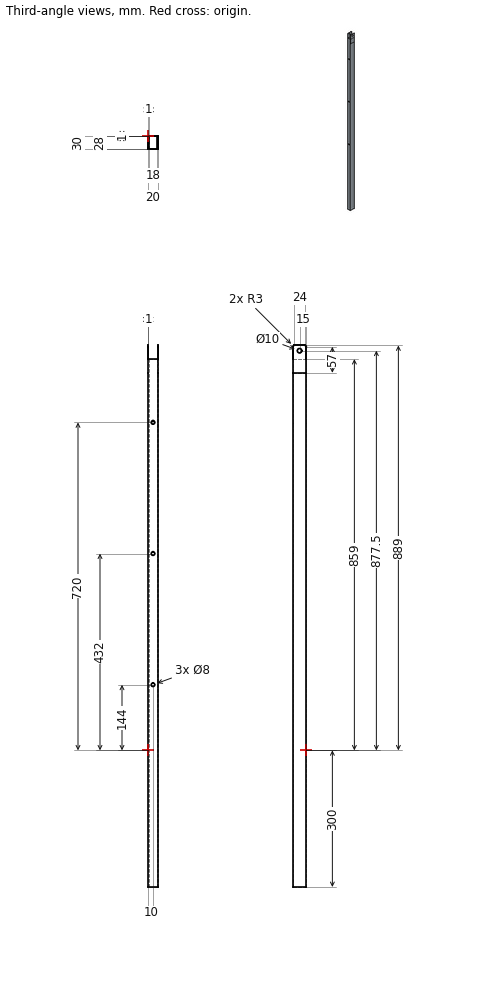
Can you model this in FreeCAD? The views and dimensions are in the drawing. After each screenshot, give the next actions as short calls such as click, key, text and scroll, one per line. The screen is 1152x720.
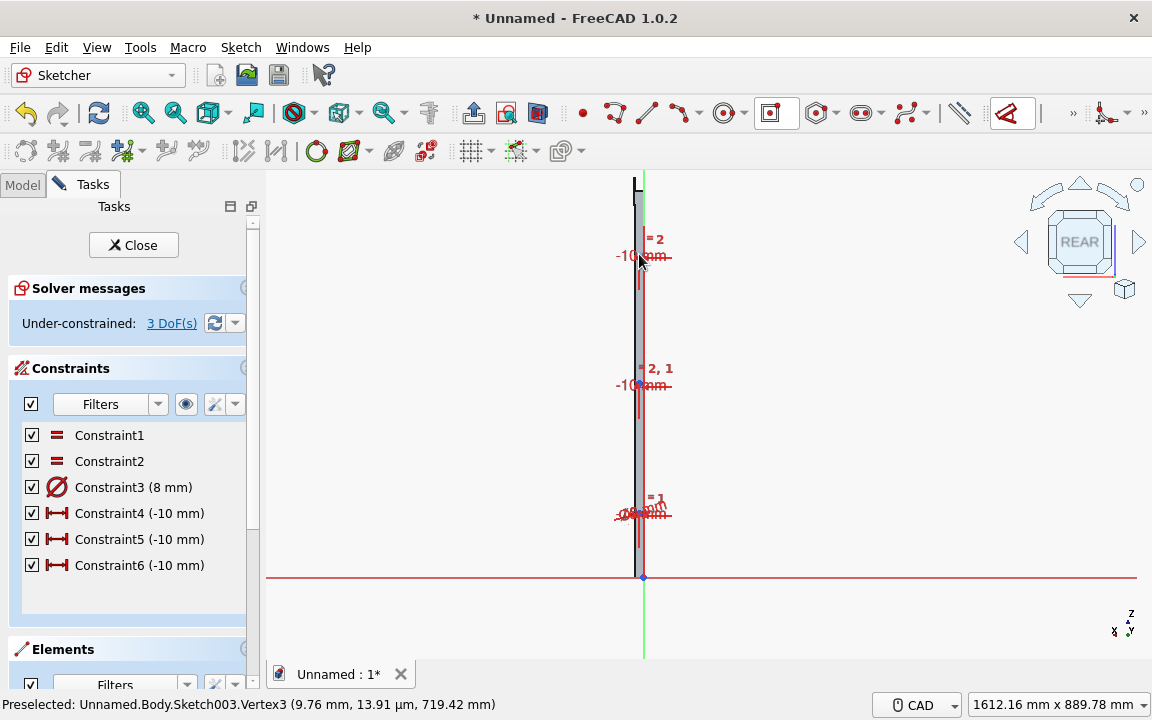
click(639, 513)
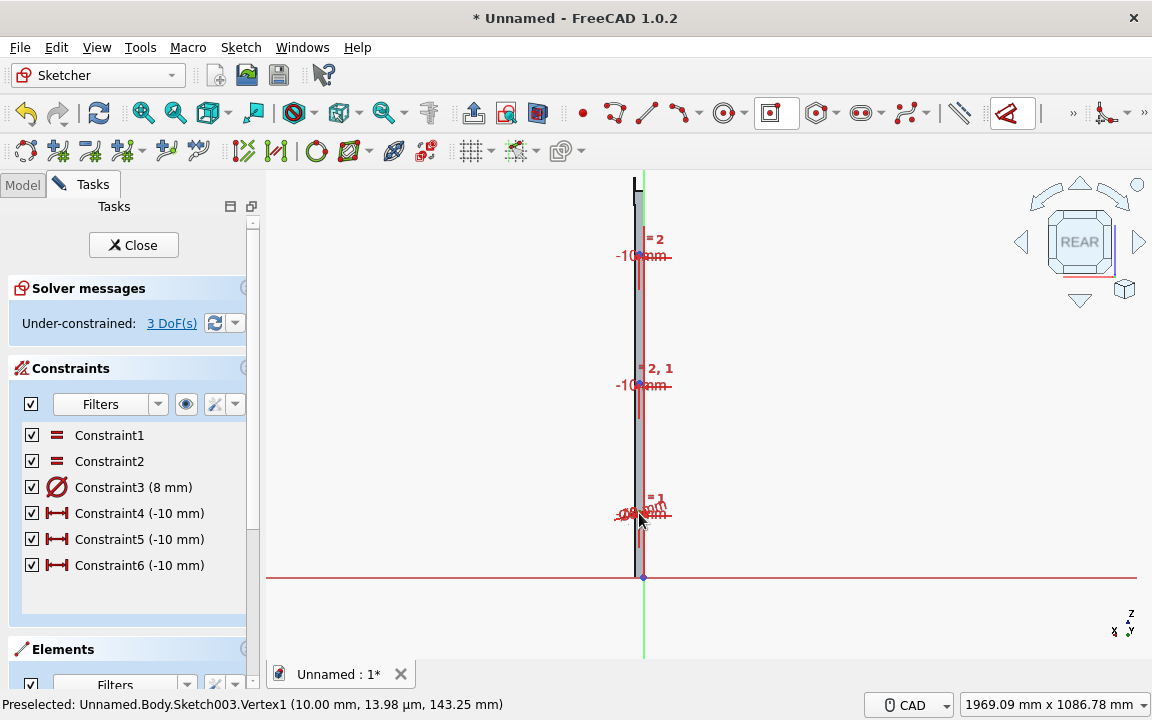
key(i)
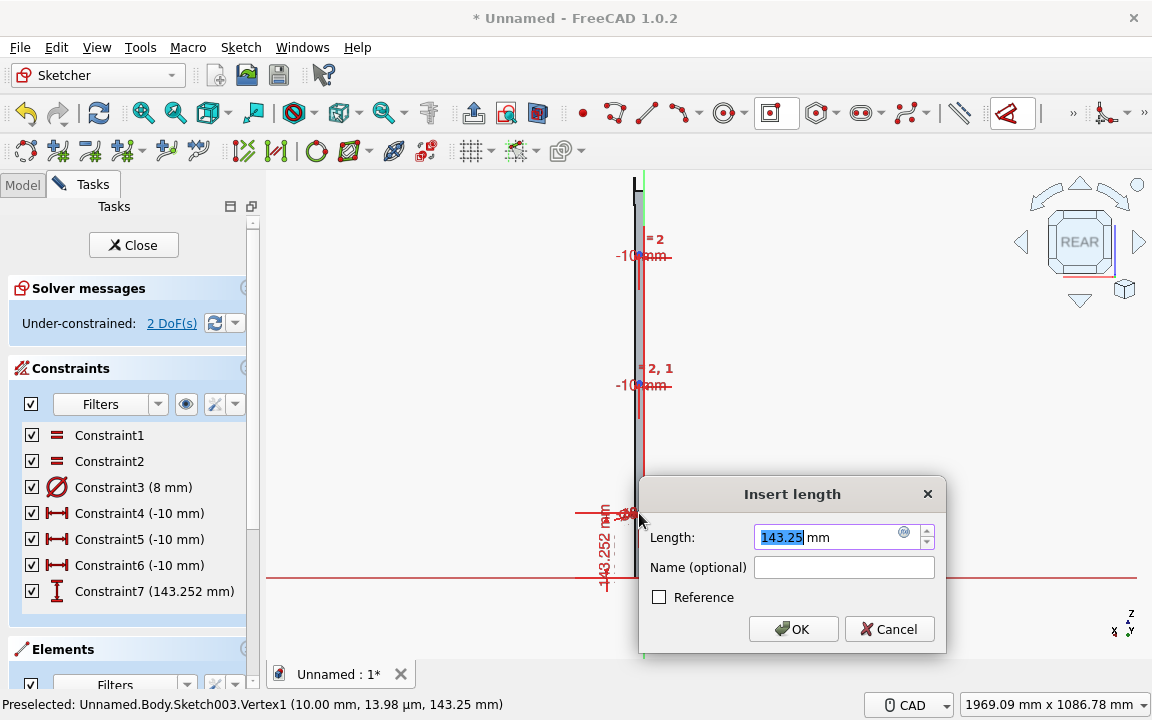
text(144)
key(Return)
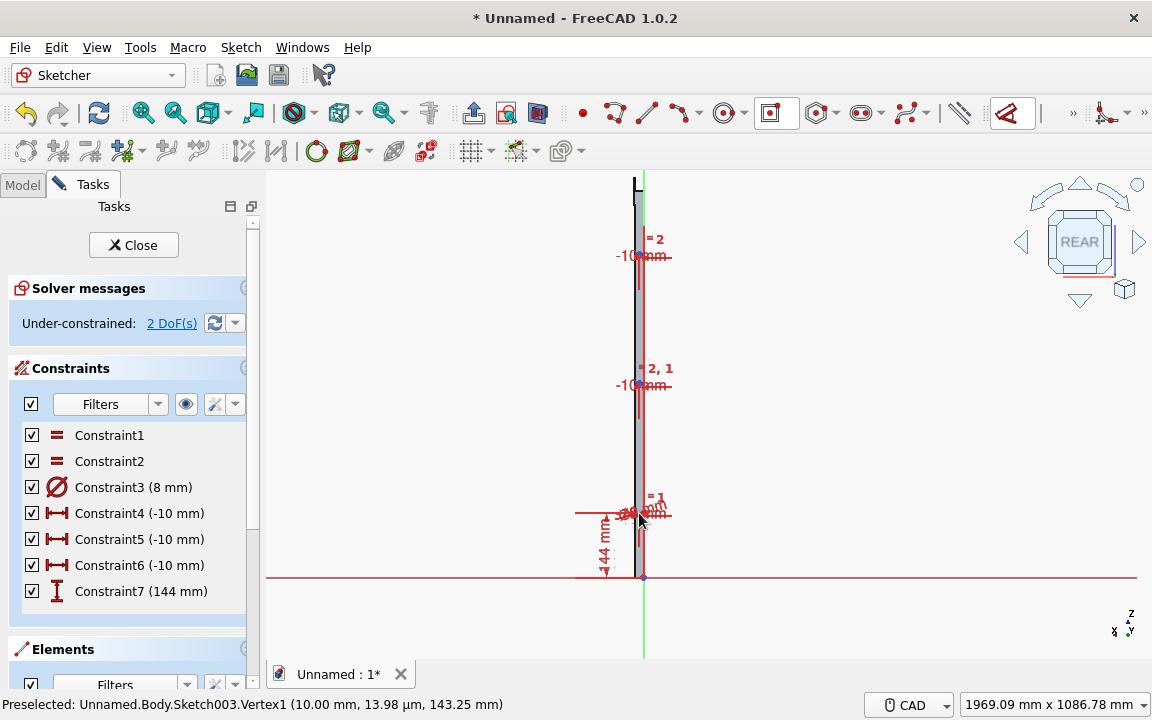
click(639, 384)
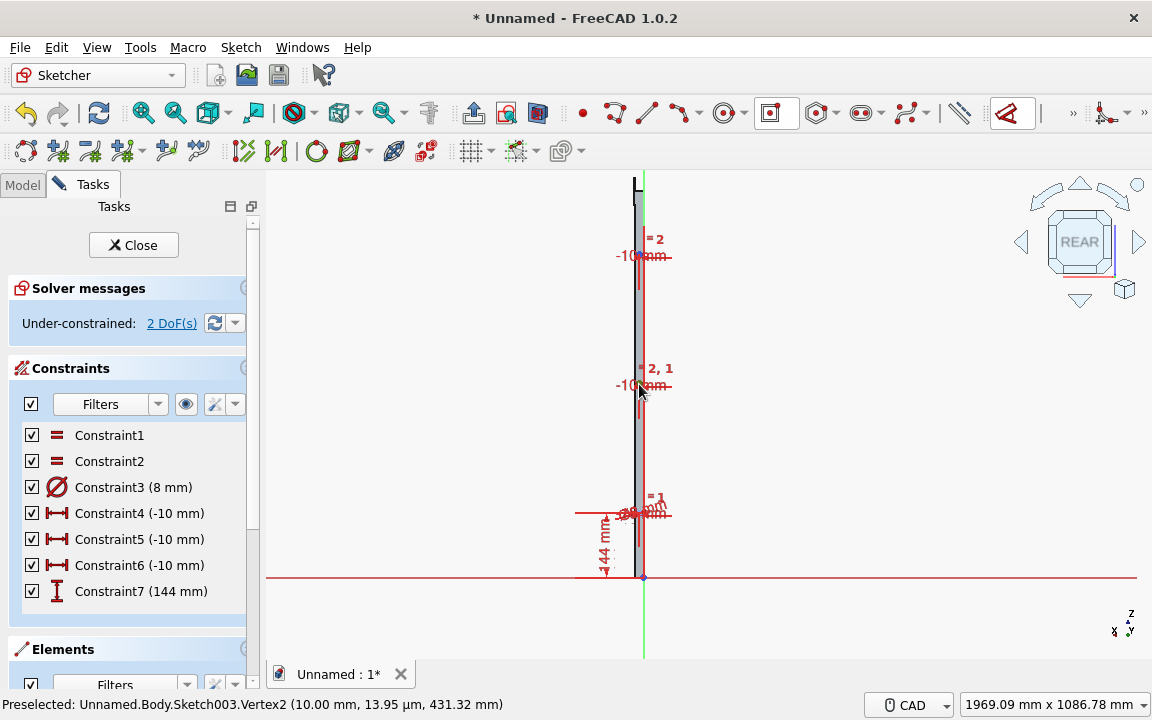
key(i)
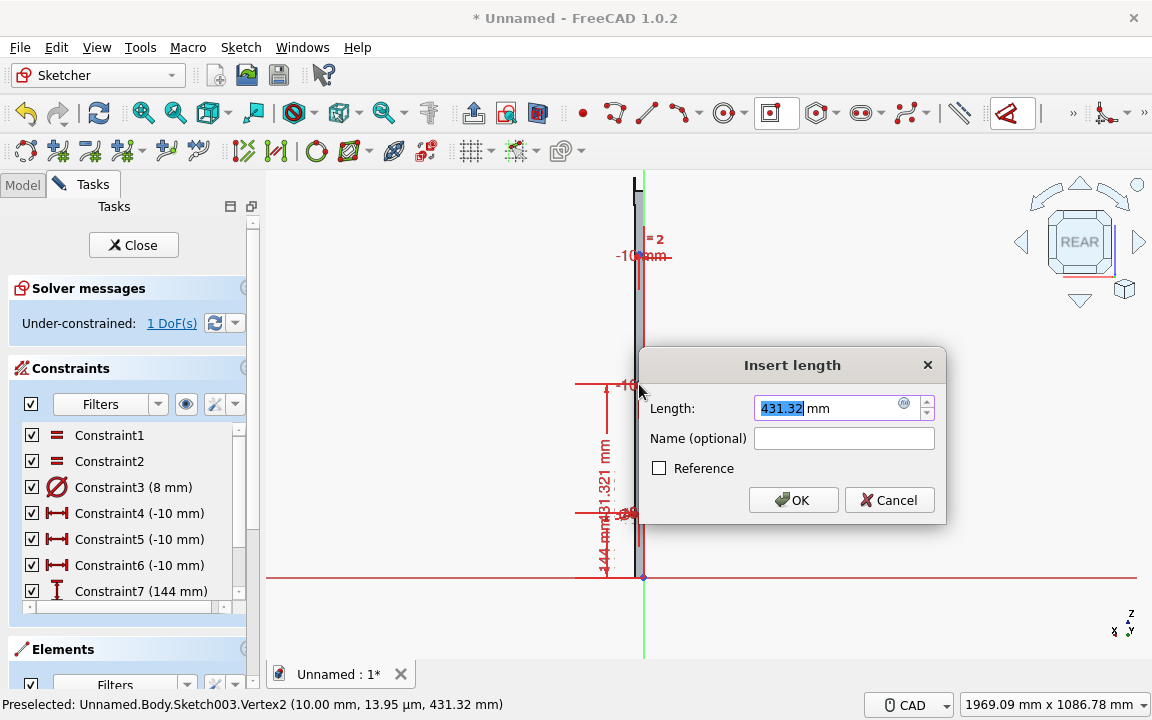
text(432)
key(Return)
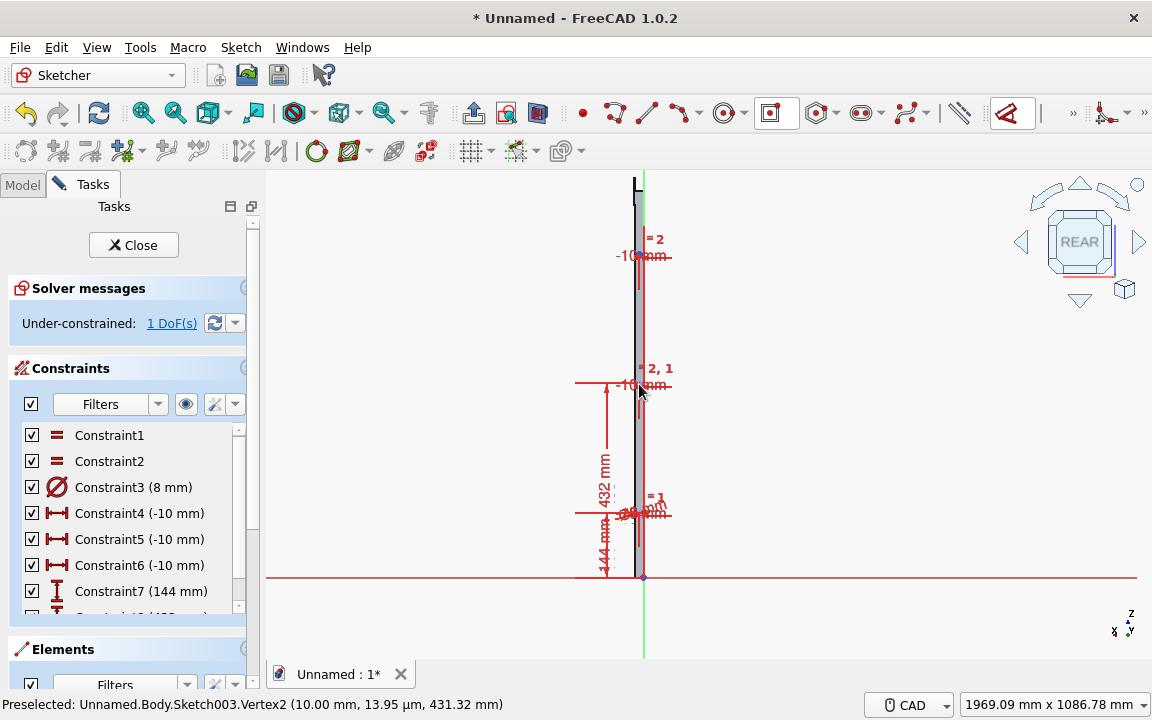
click(639, 254)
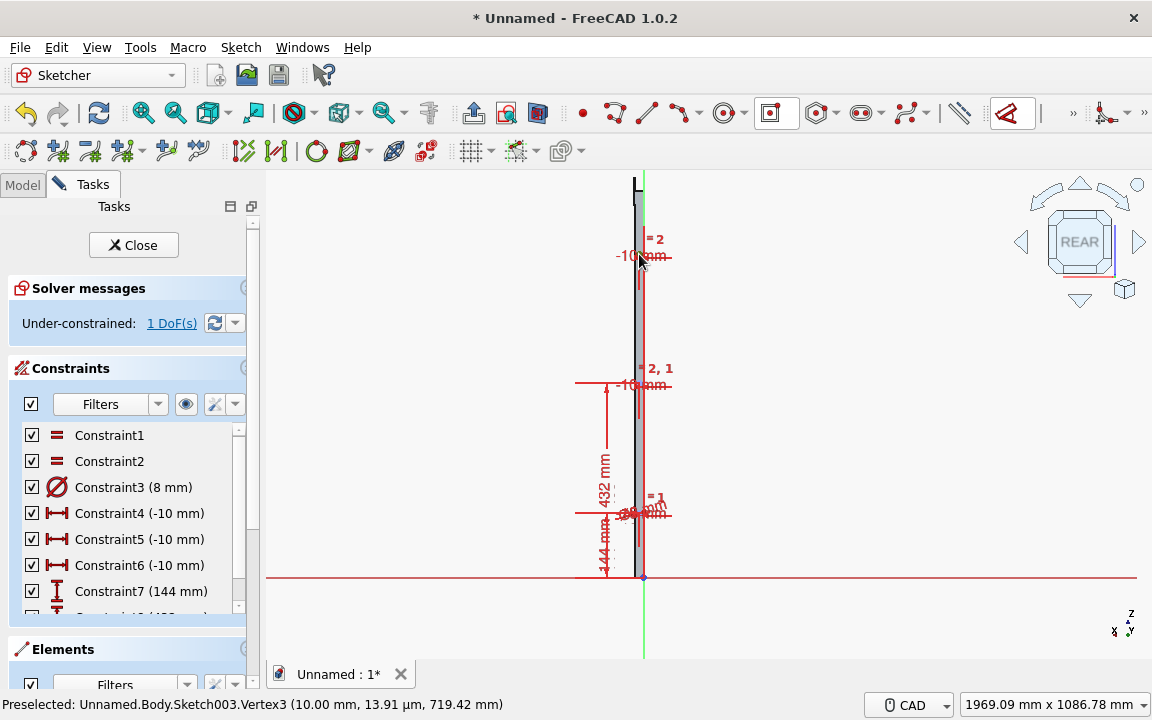
key(i)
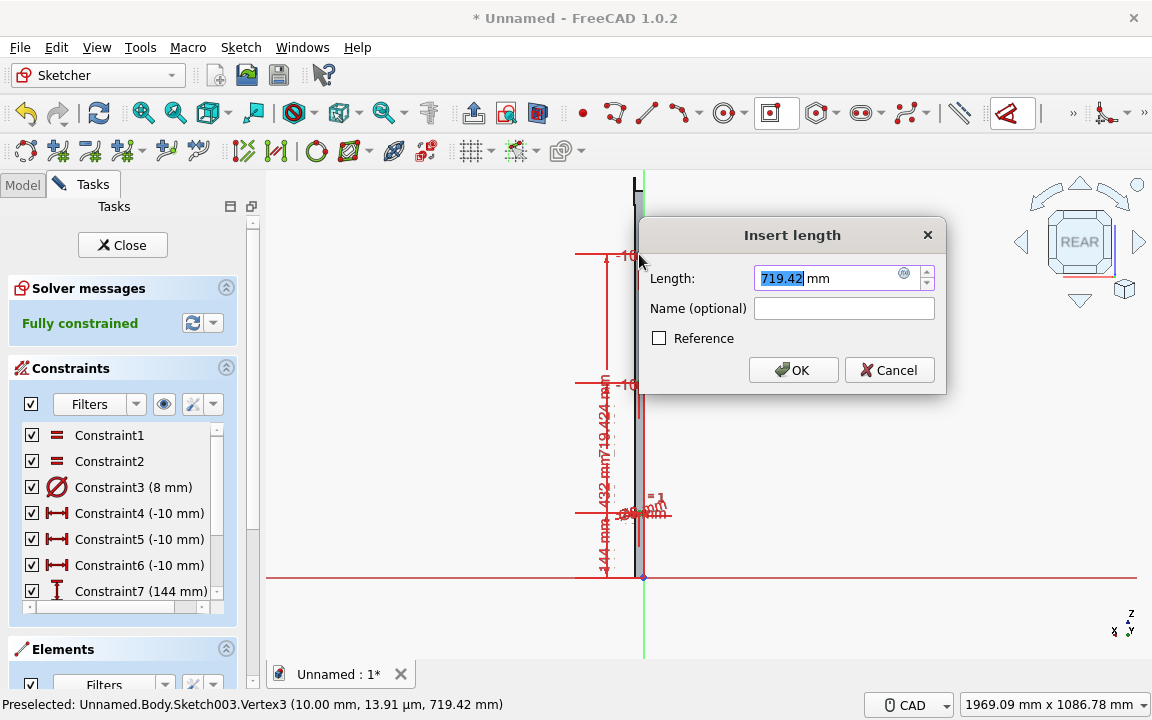
text(720)
key(Return)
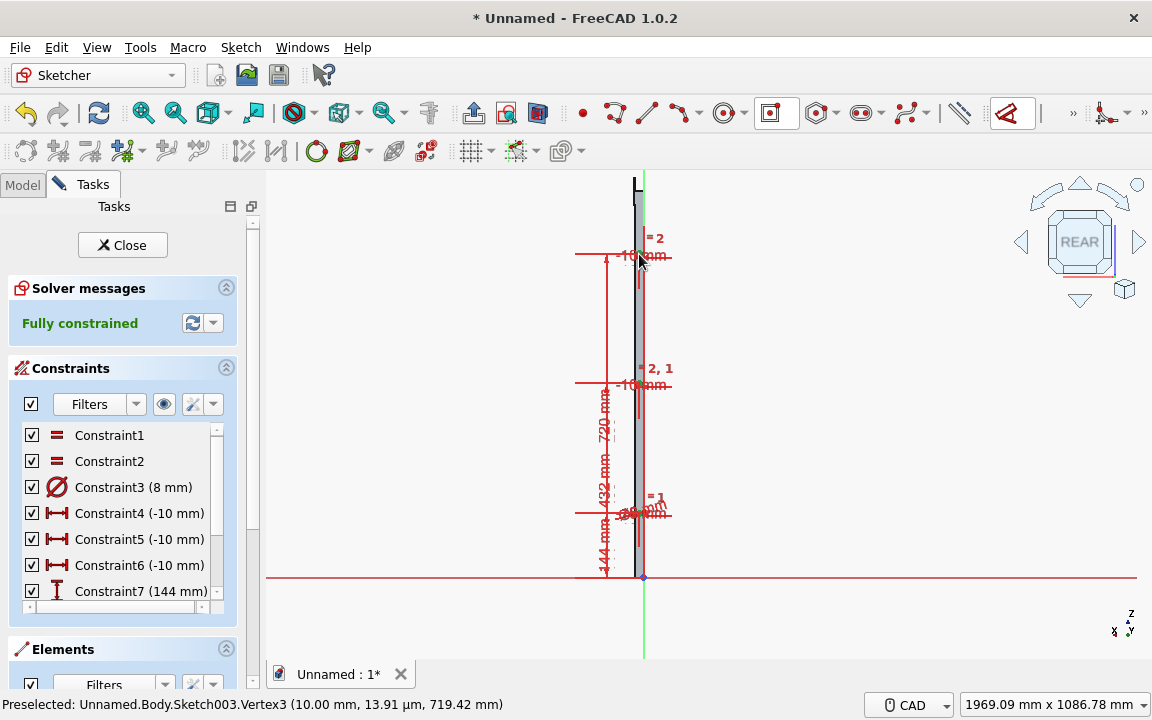
click(123, 245)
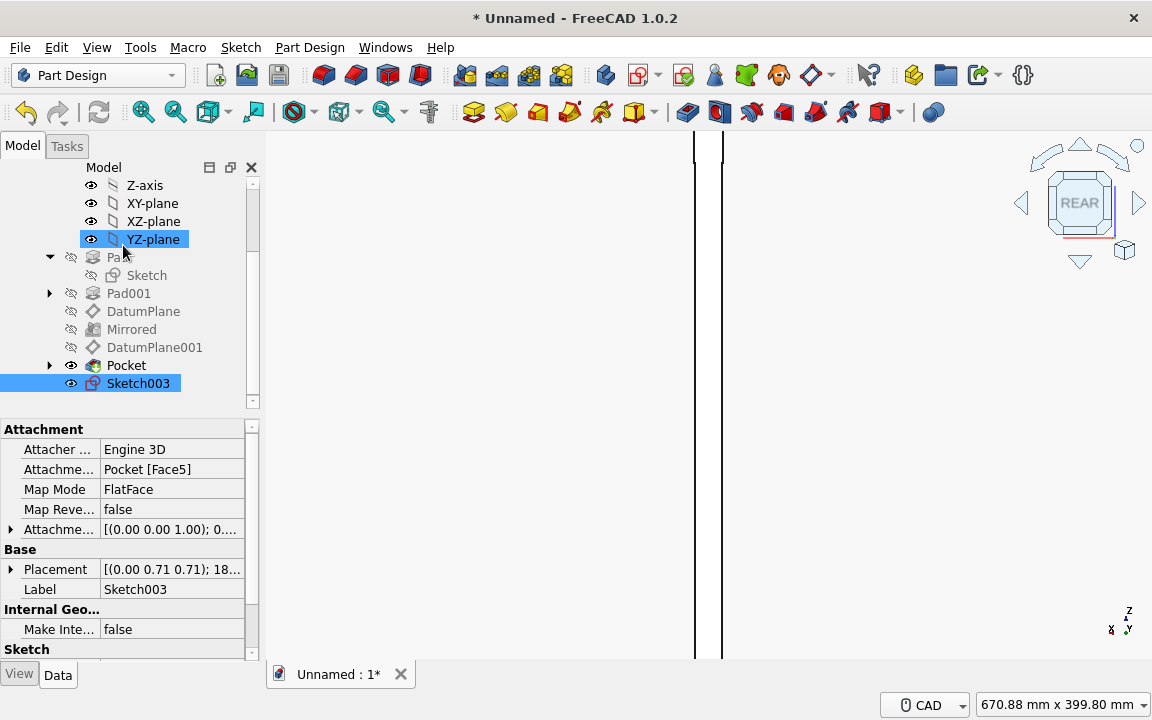
click(688, 112)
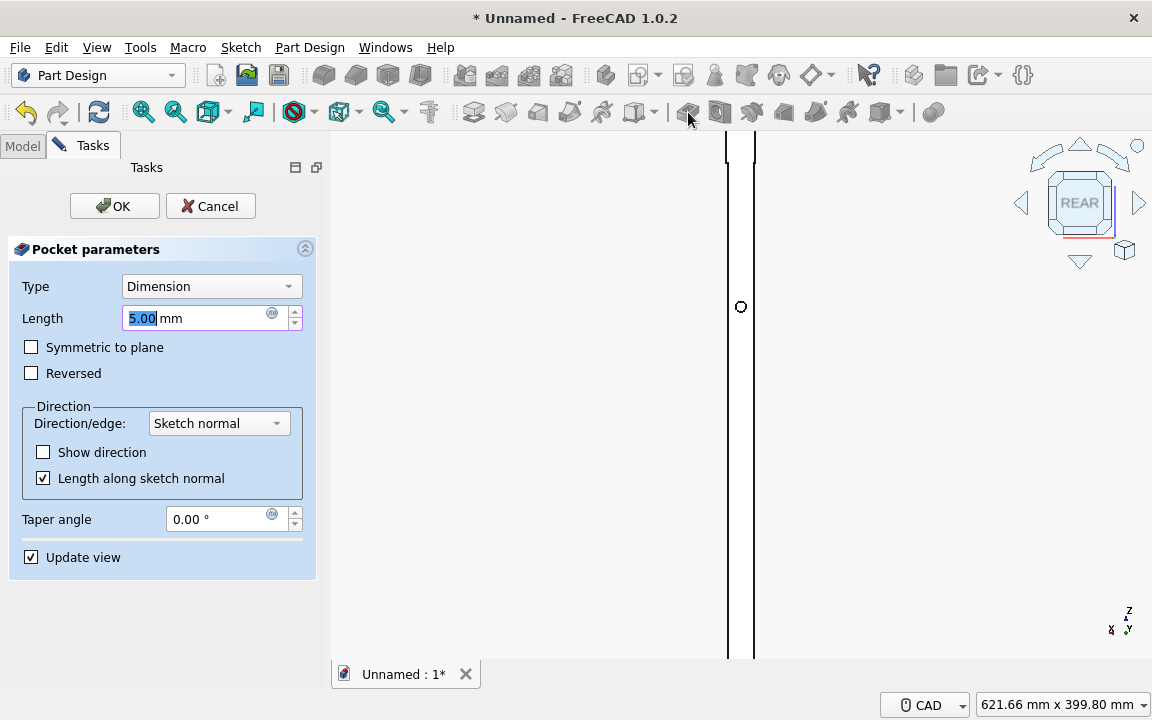
click(212, 286)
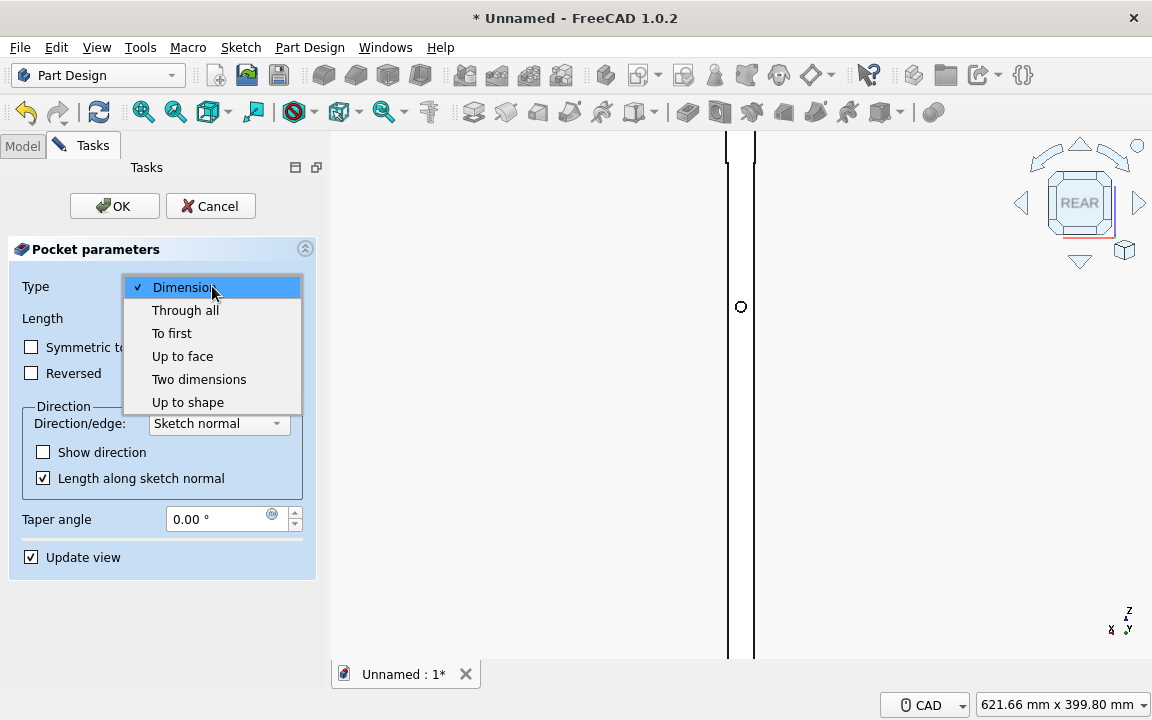
click(212, 310)